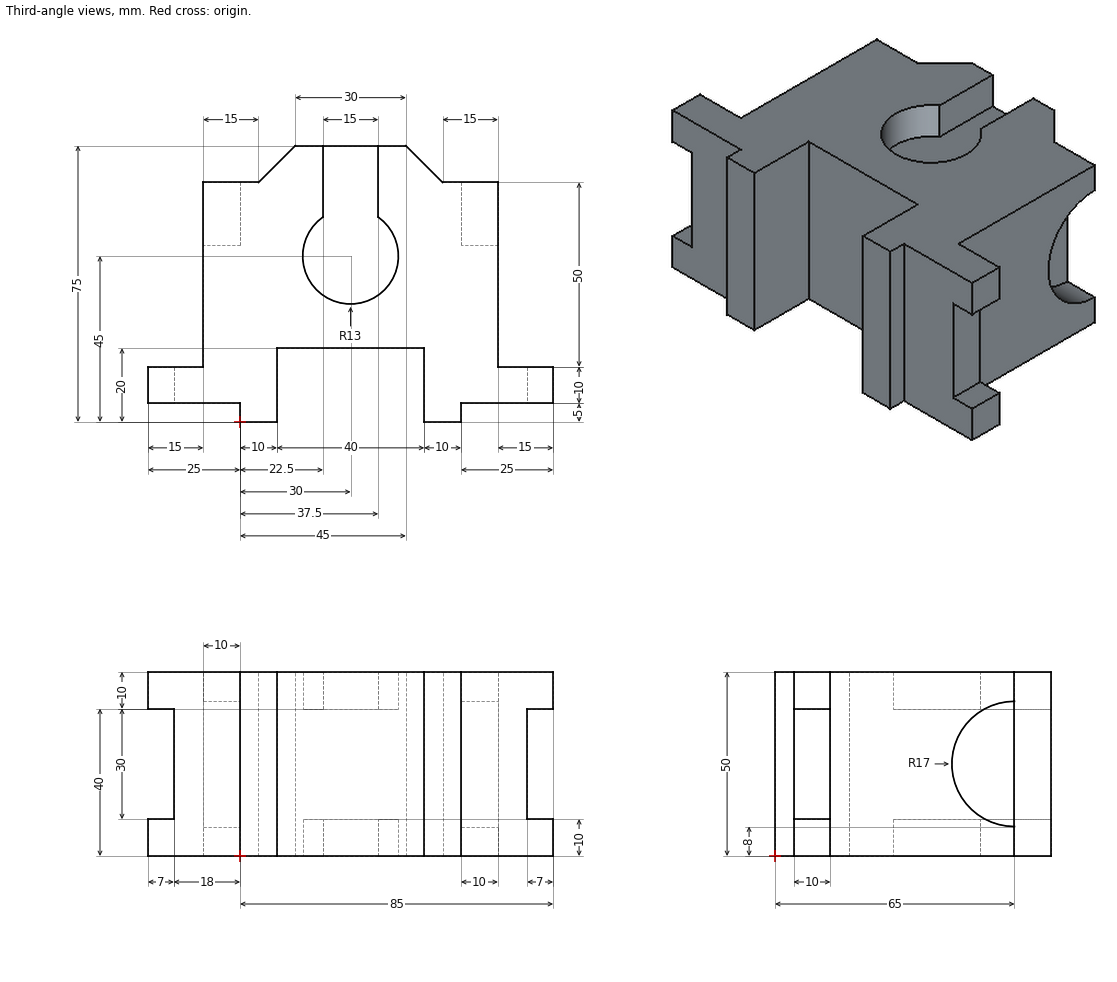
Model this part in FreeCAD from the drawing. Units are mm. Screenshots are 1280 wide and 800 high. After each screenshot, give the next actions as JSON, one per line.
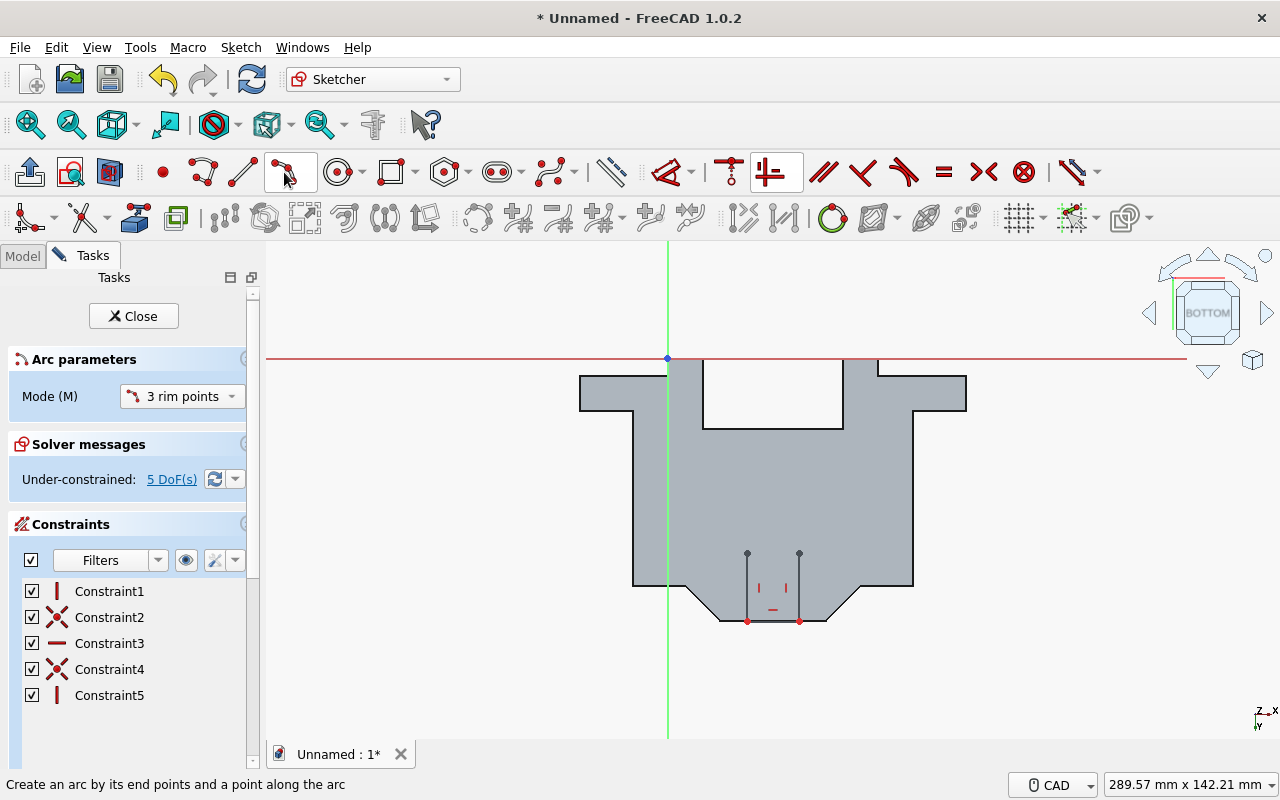
{"action": "left_click", "coordinate": [799, 554]}
{"action": "left_click", "coordinate": [747, 554]}
{"action": "left_click", "coordinate": [773, 471]}
{"action": "key", "text": "Escape"}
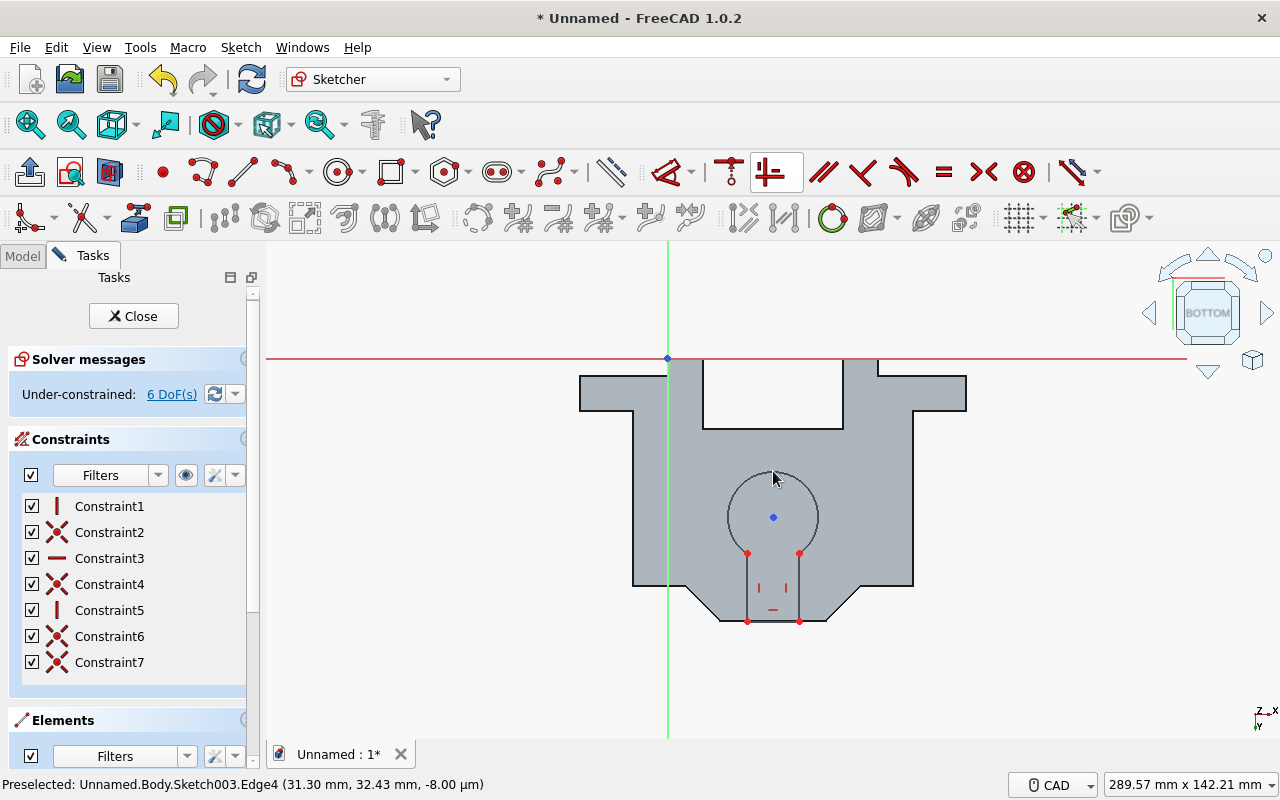
{"action": "left_click", "coordinate": [666, 172]}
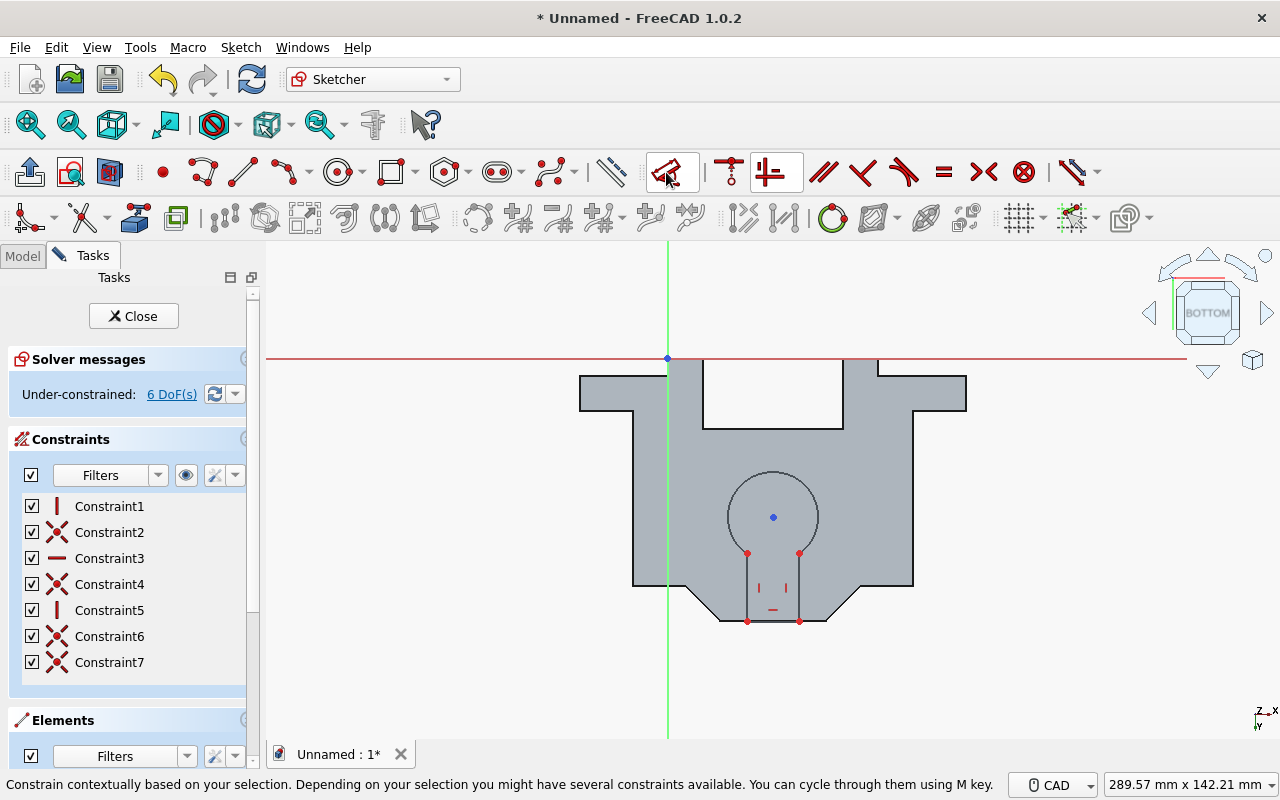
{"action": "left_click", "coordinate": [811, 493]}
{"action": "left_click", "coordinate": [838, 476]}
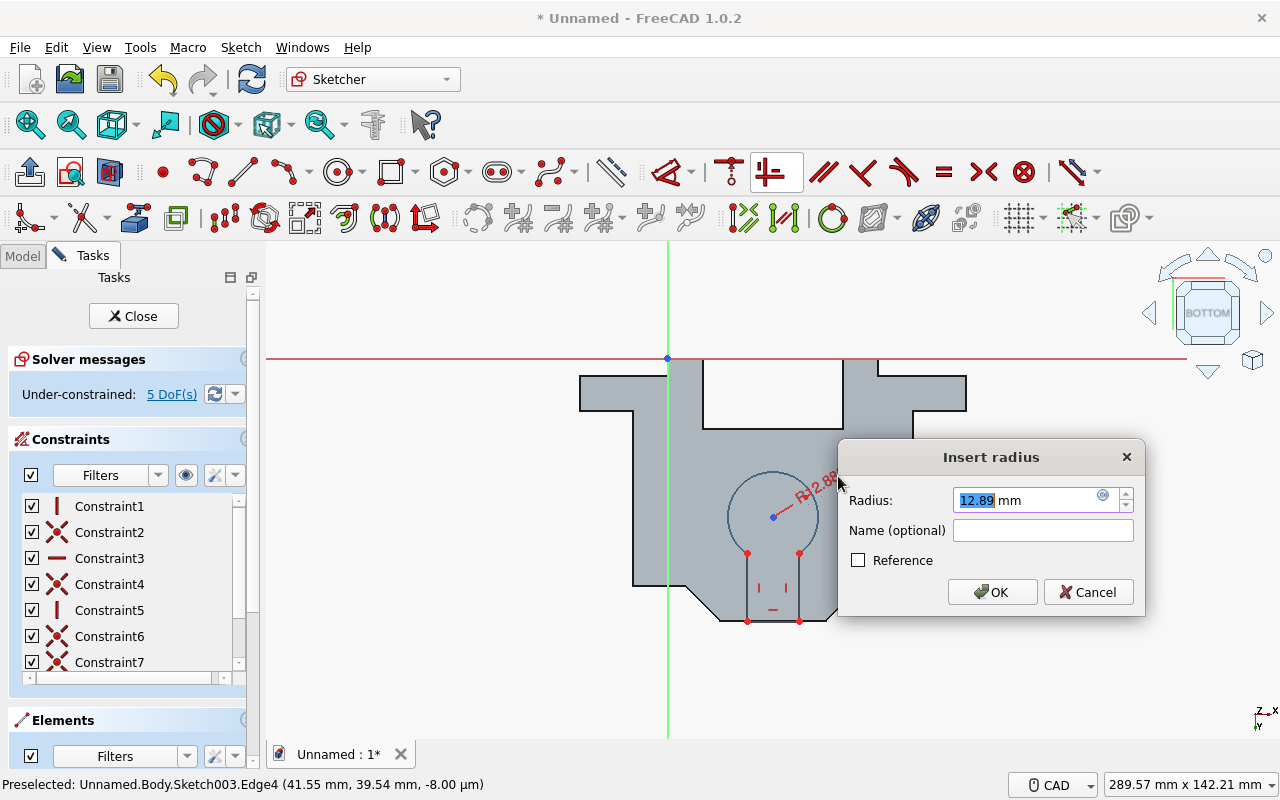
{"action": "type", "text": "13"}
{"action": "key", "text": "Return"}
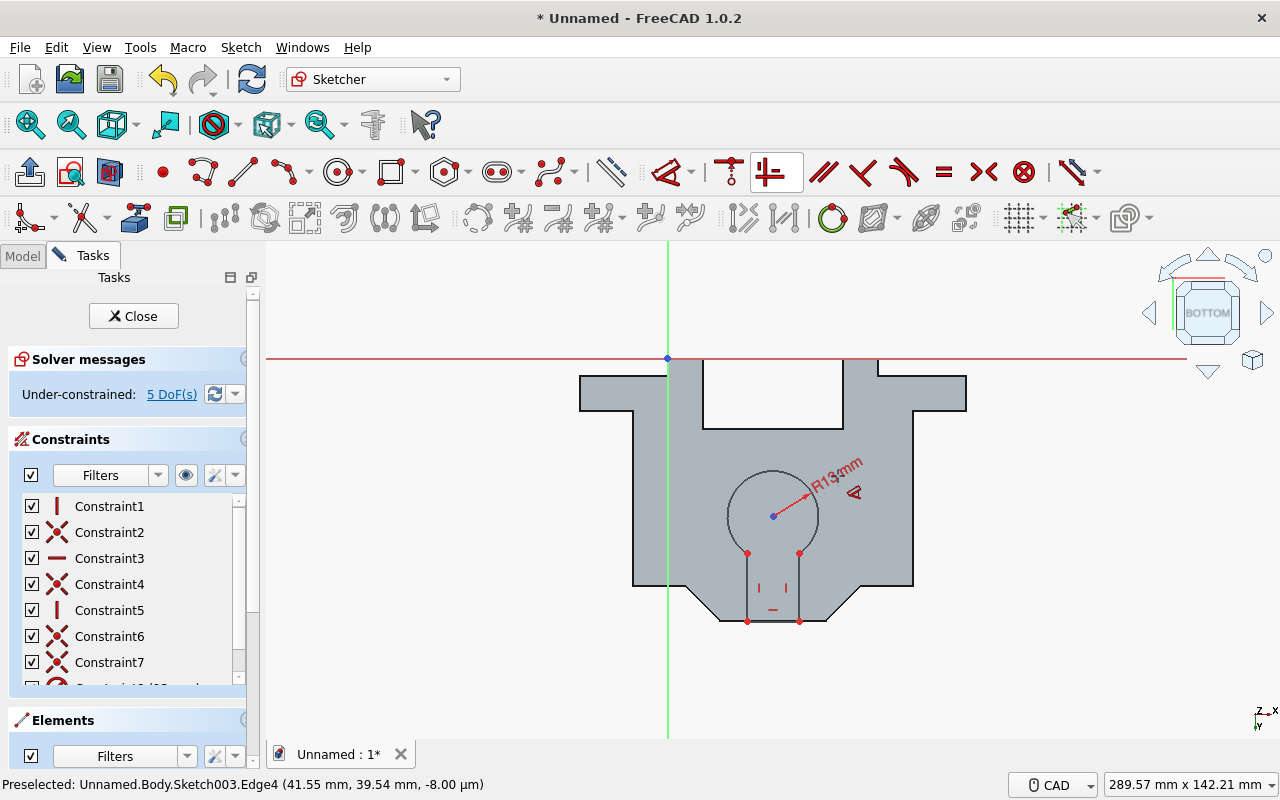
{"action": "left_click", "coordinate": [763, 622]}
{"action": "left_click", "coordinate": [773, 656]}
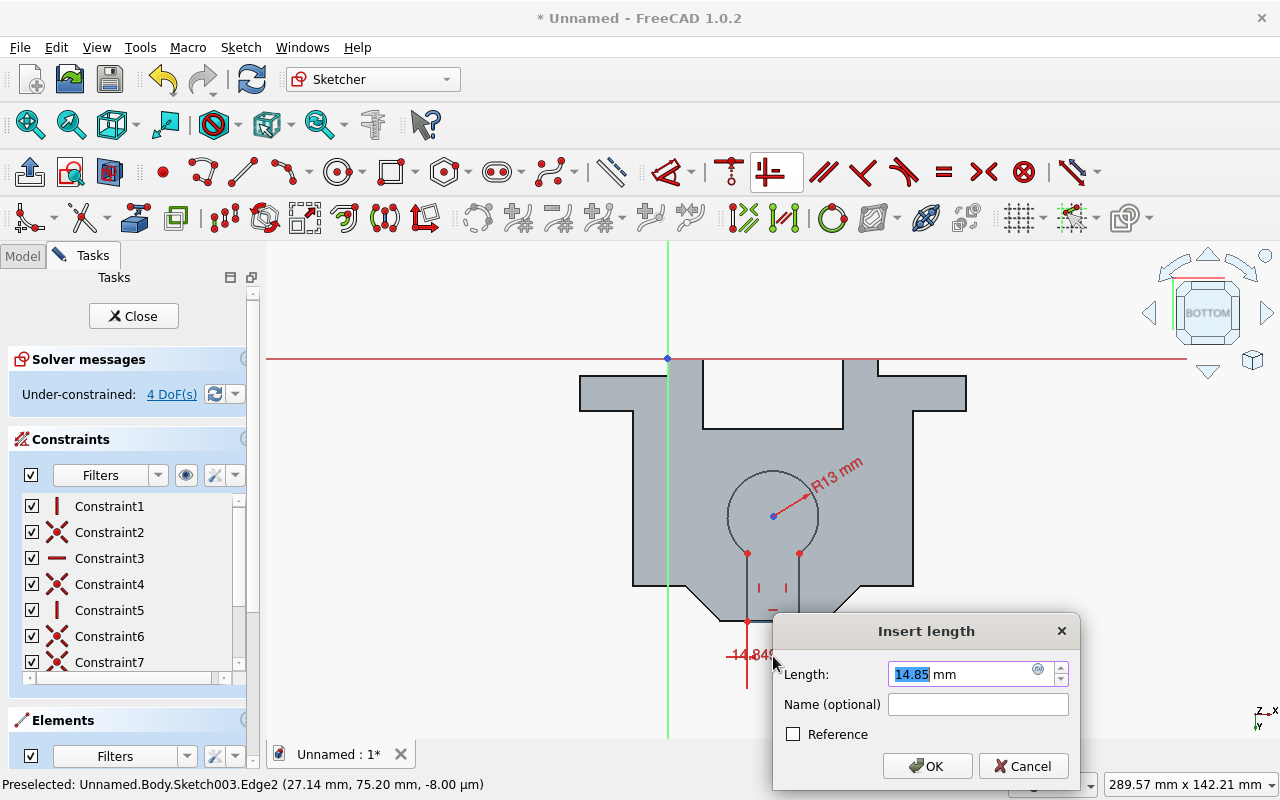
{"action": "type", "text": "15"}
{"action": "key", "text": "Return"}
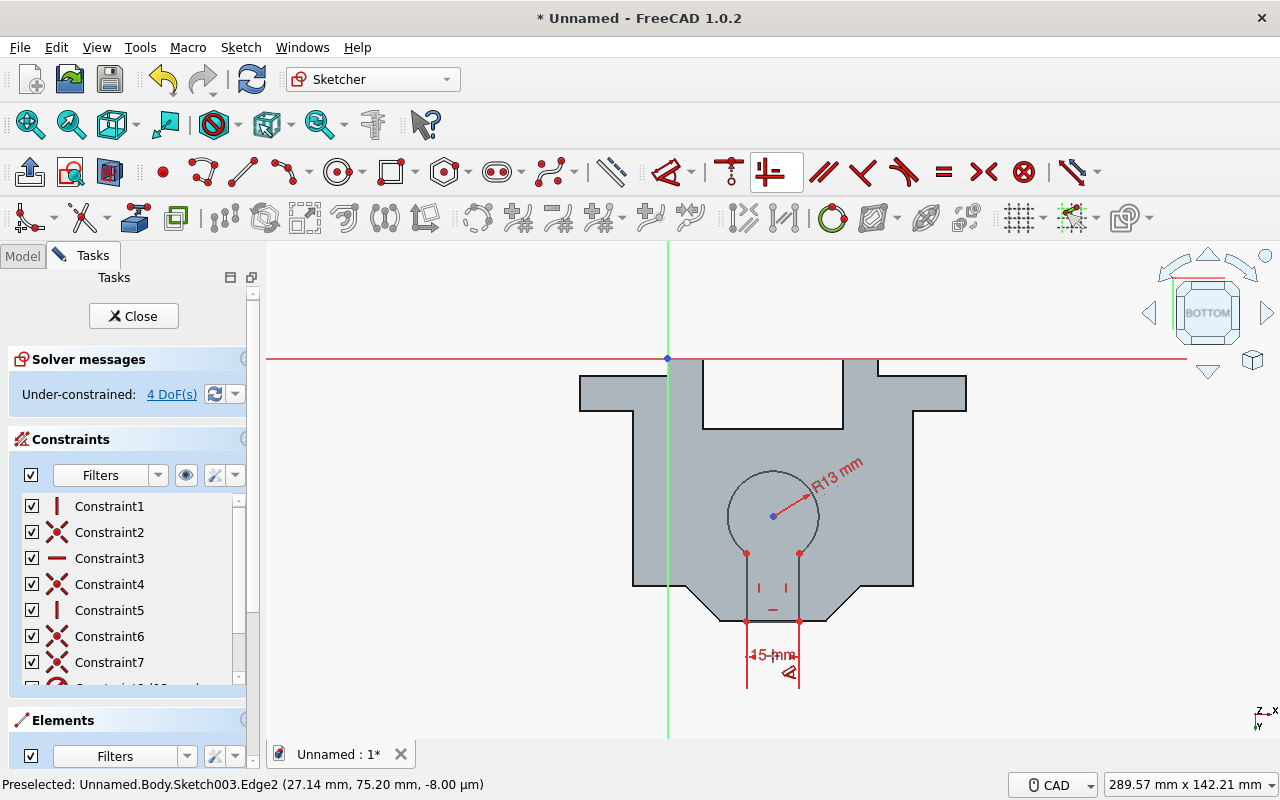
{"action": "left_click", "coordinate": [747, 622]}
{"action": "left_click", "coordinate": [634, 490]}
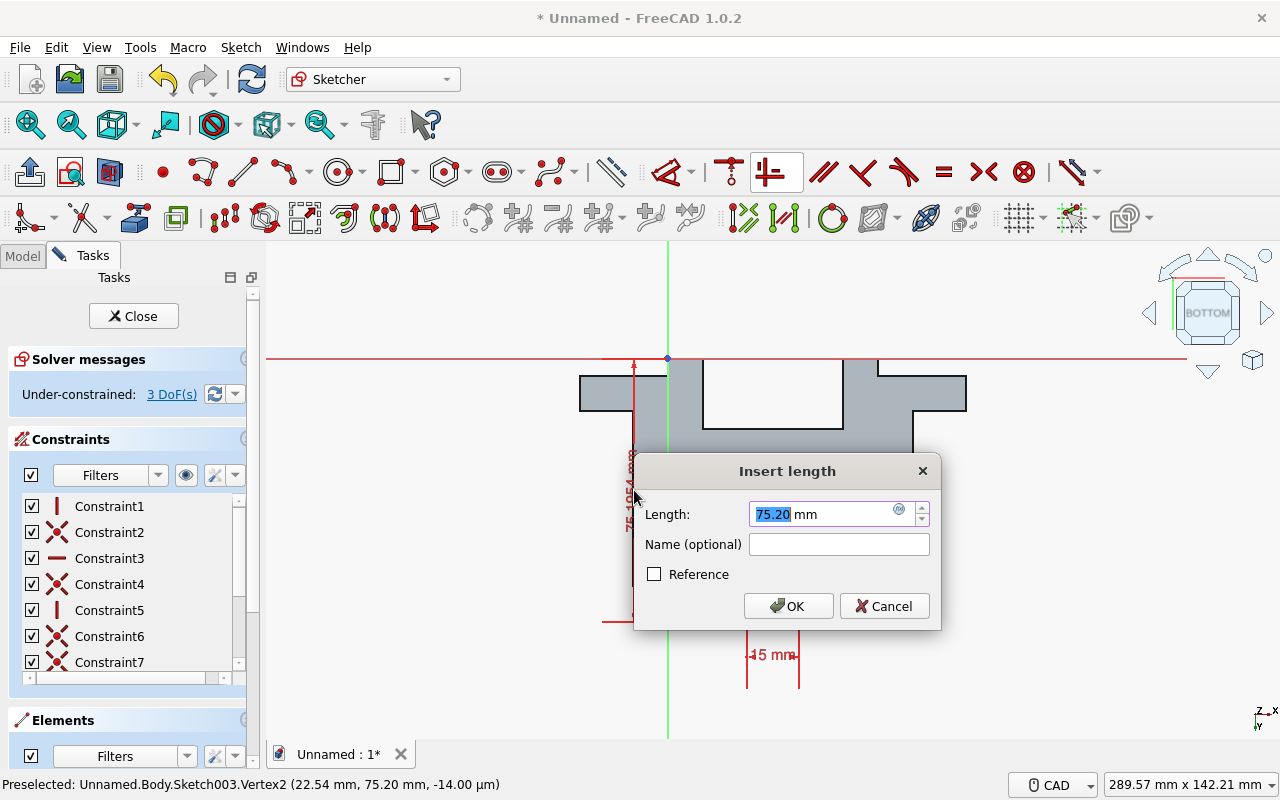
{"action": "type", "text": "75"}
{"action": "key", "text": "Return"}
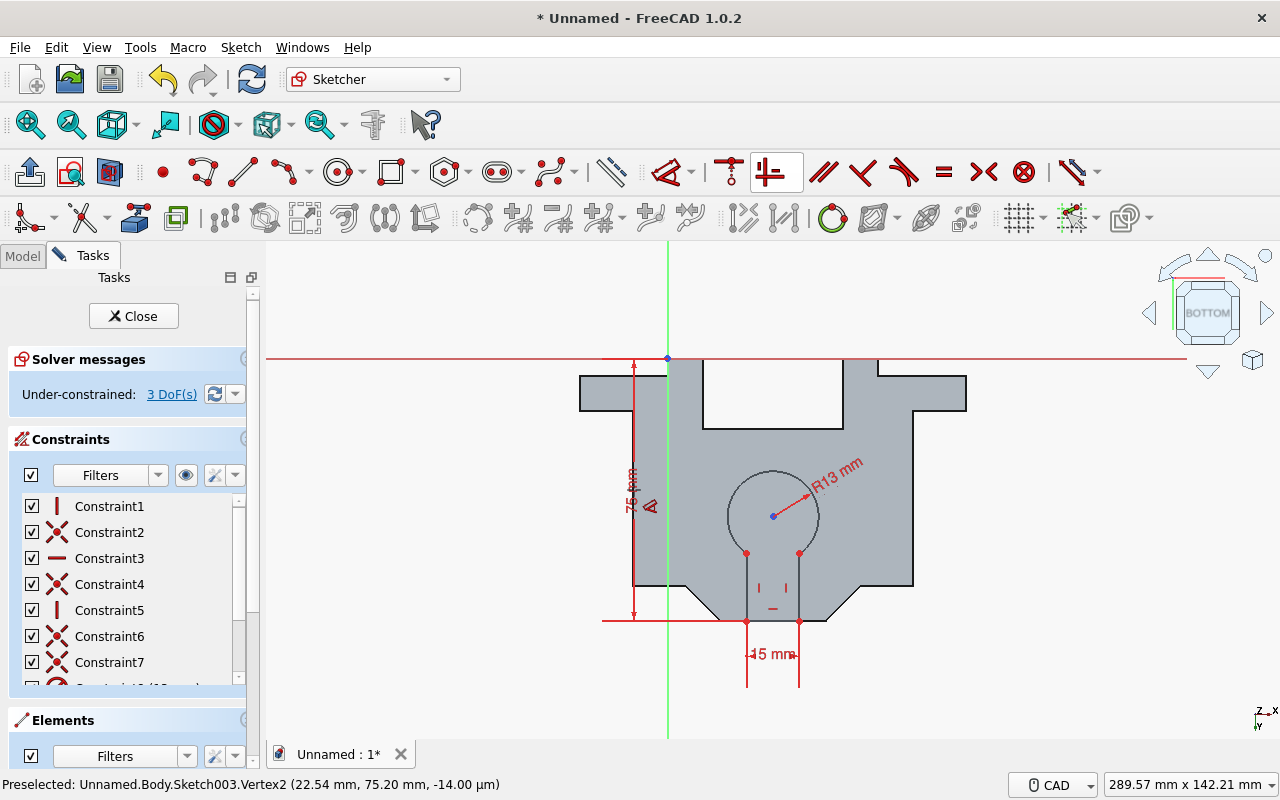
{"action": "left_click", "coordinate": [773, 517]}
{"action": "left_click", "coordinate": [721, 325]}